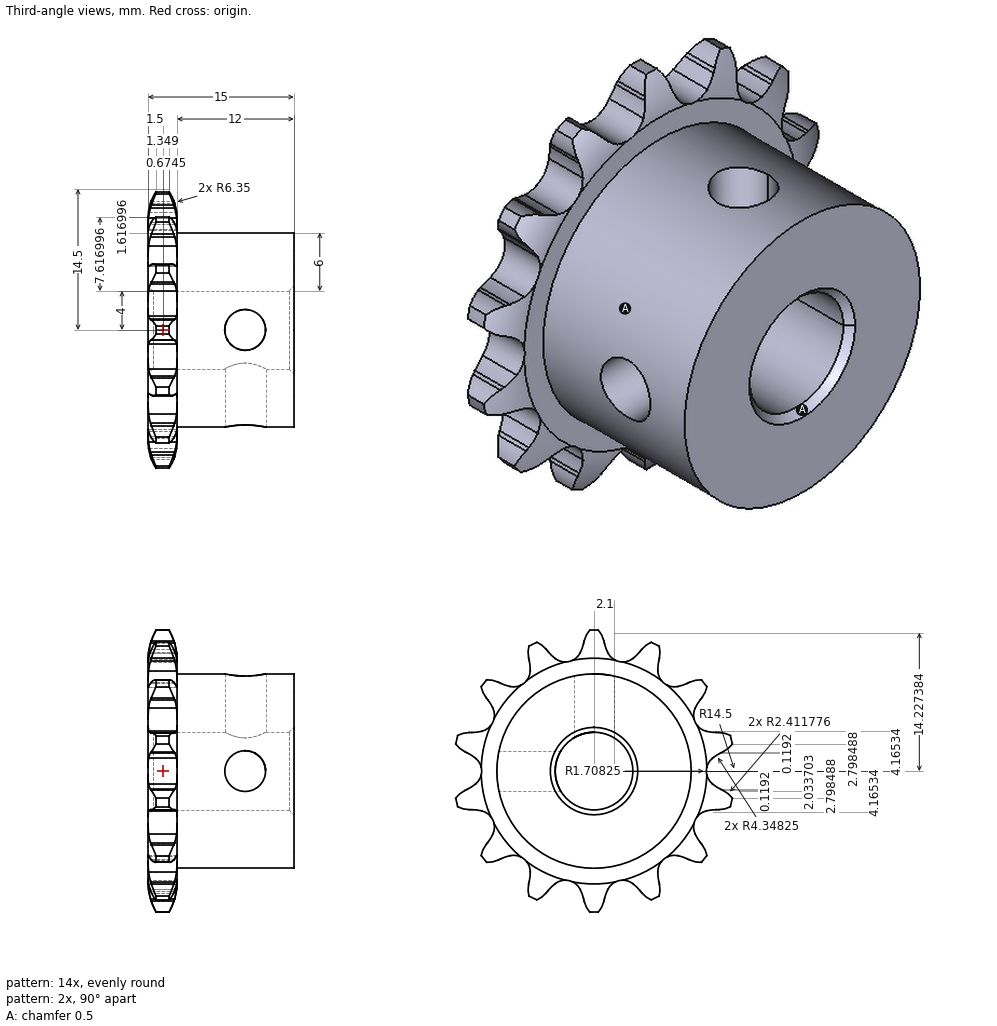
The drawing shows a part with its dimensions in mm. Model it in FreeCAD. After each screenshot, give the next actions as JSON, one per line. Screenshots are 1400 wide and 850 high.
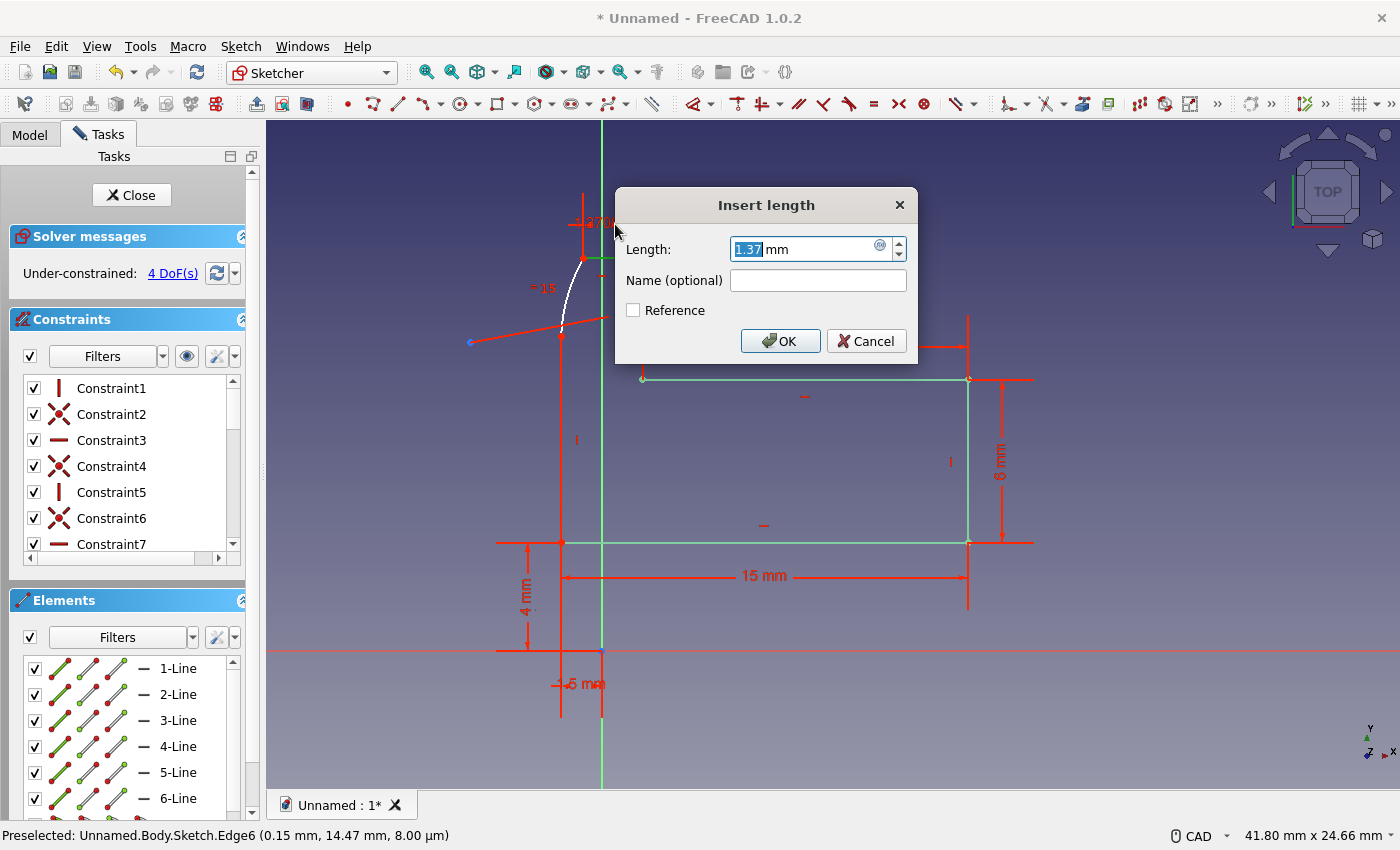
{"action": "type", "text": "1.349"}
{"action": "key", "text": "Return"}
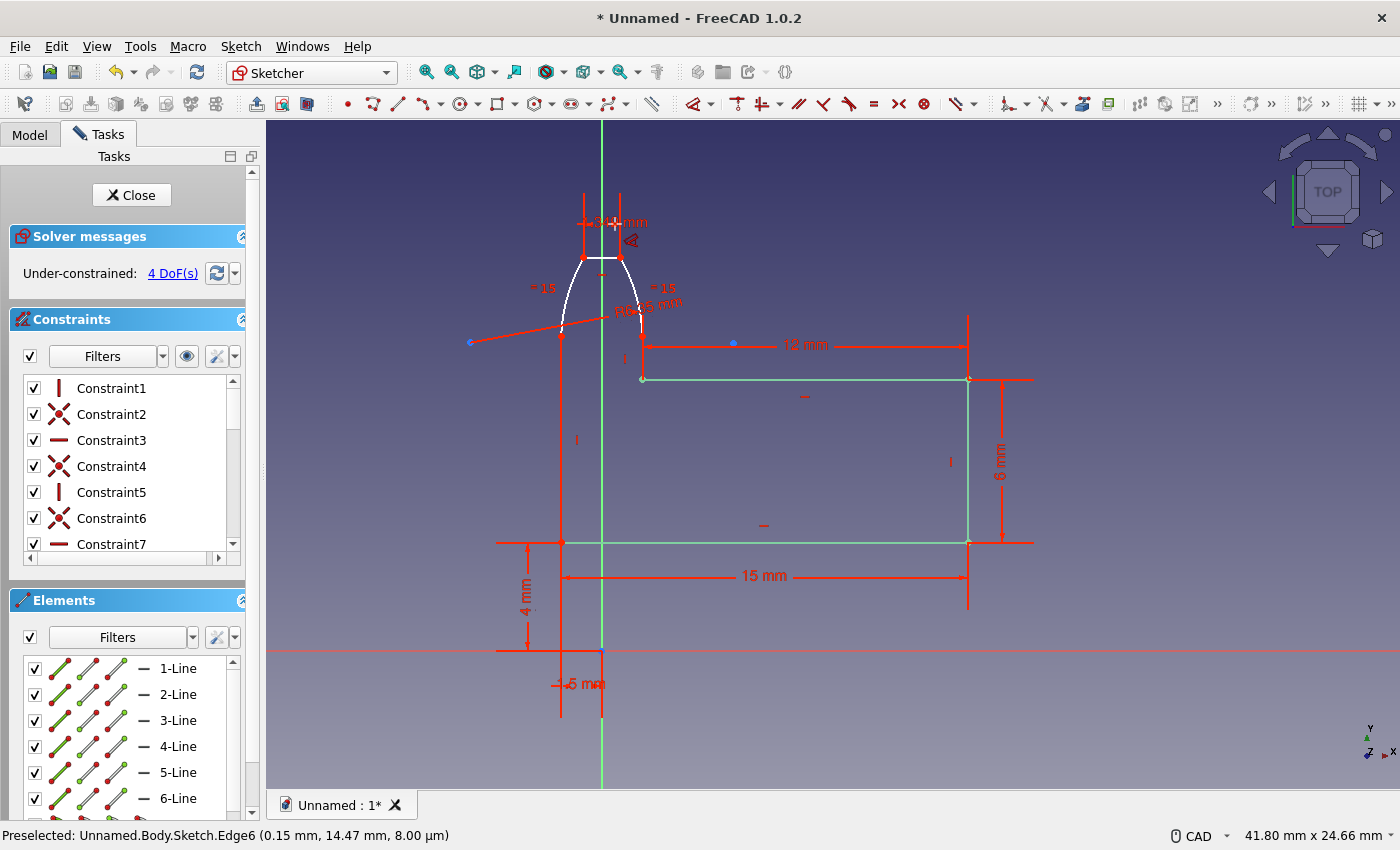
{"action": "left_click", "coordinate": [620, 258]}
{"action": "left_click", "coordinate": [654, 454]}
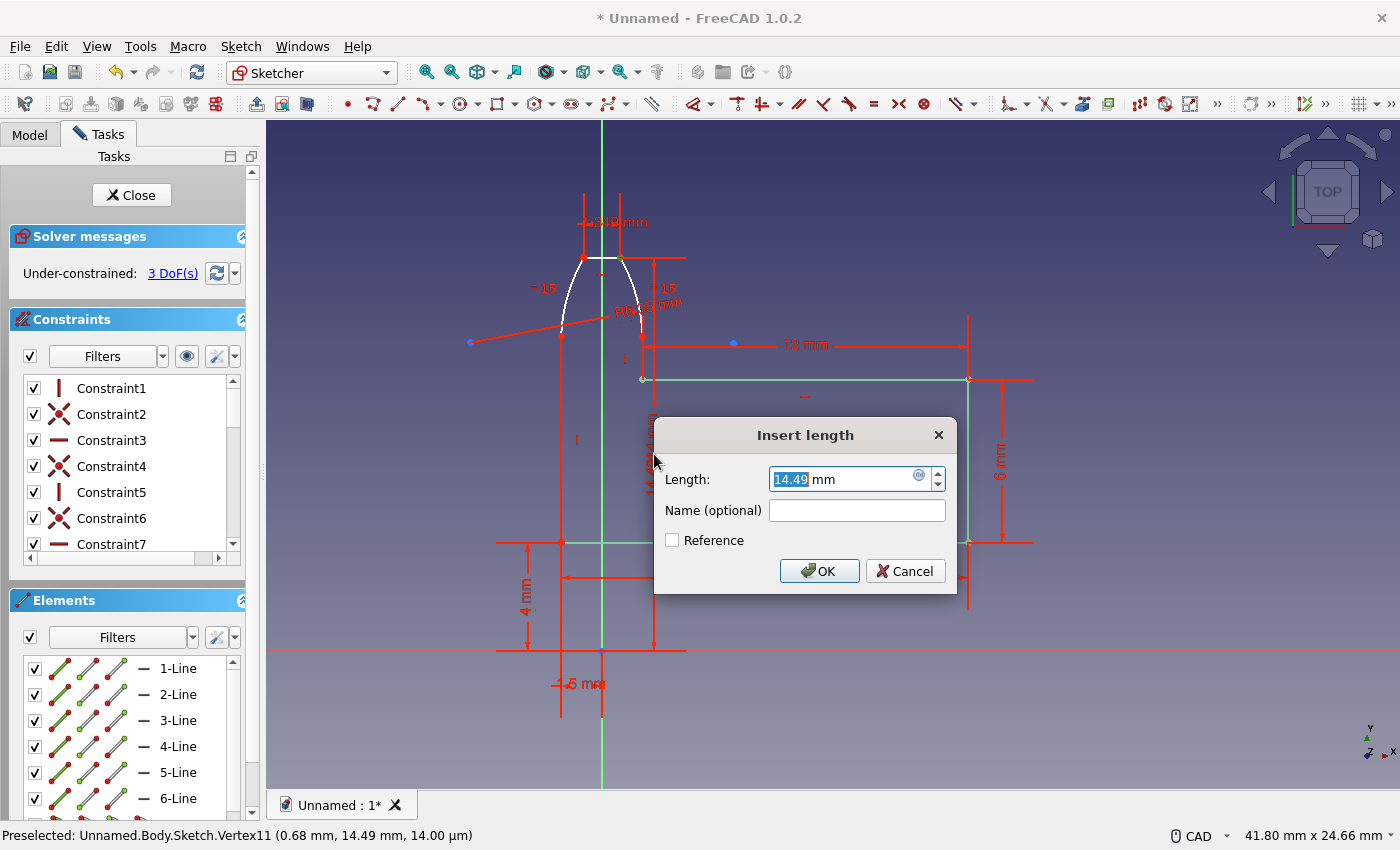
{"action": "type", "text": "14.5"}
{"action": "key", "text": "Return"}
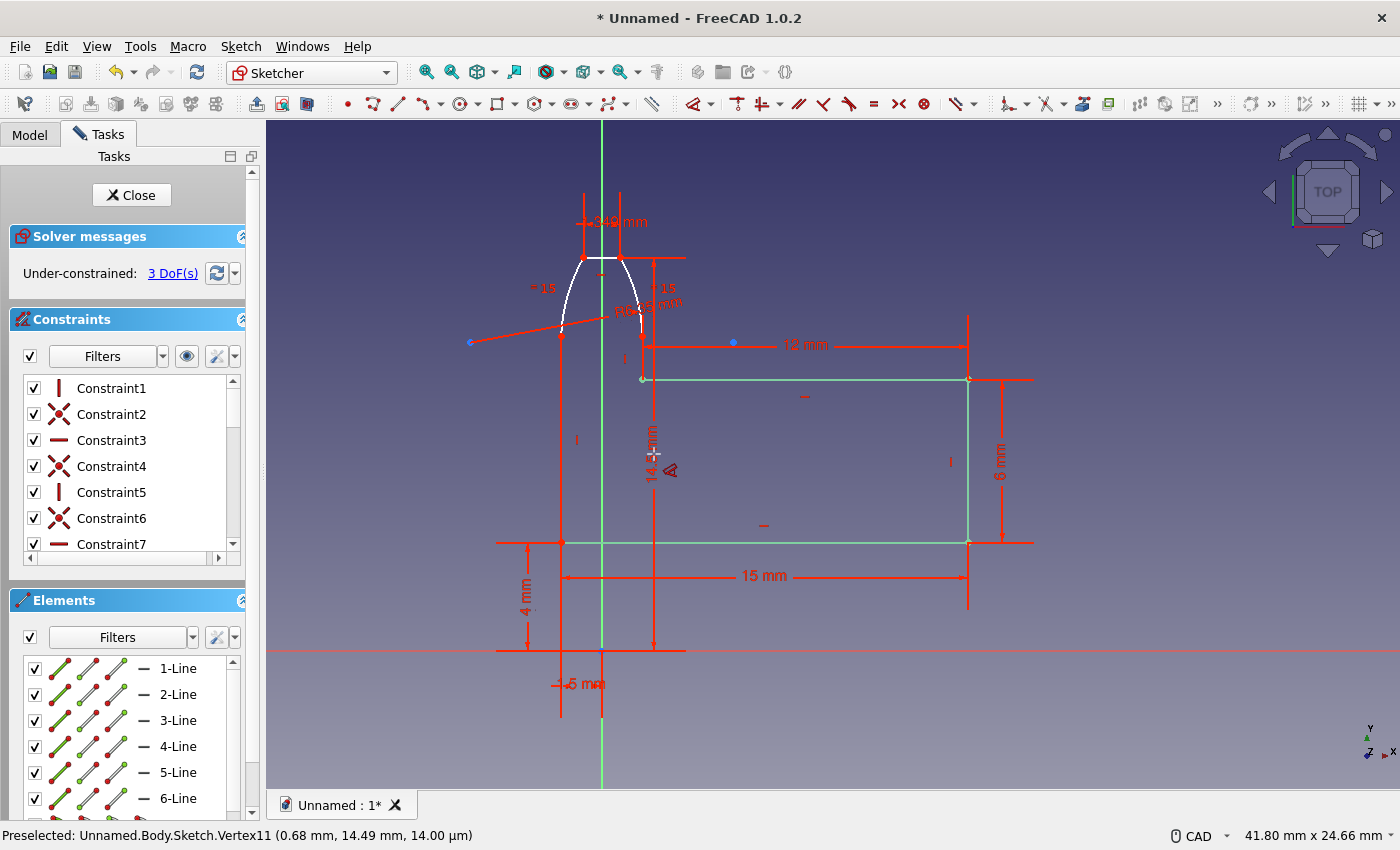
{"action": "scroll", "coordinate": [620, 258], "scroll_direction": "up", "scroll_amount": 4}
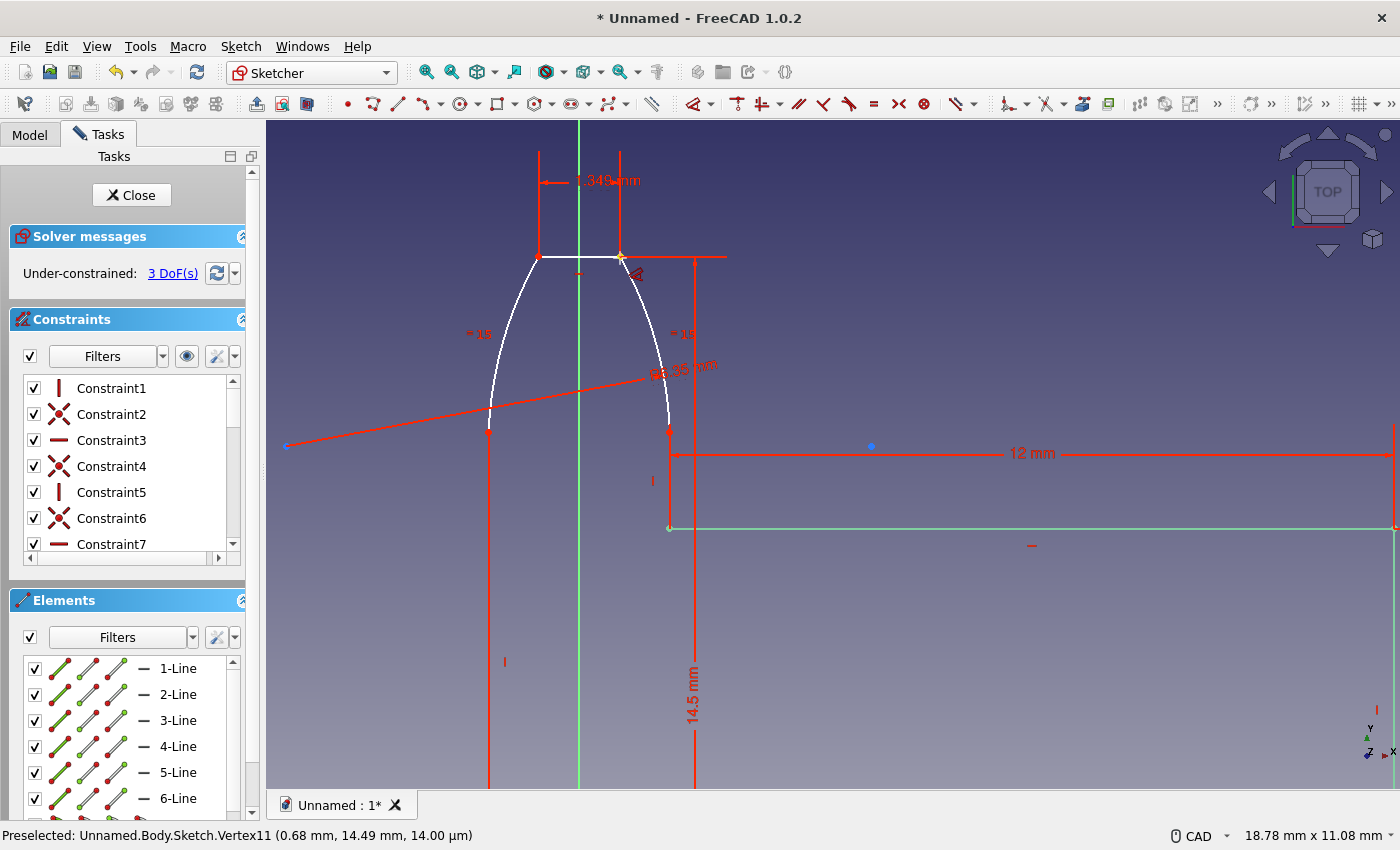
{"action": "left_click", "coordinate": [620, 257]}
{"action": "left_click", "coordinate": [600, 223]}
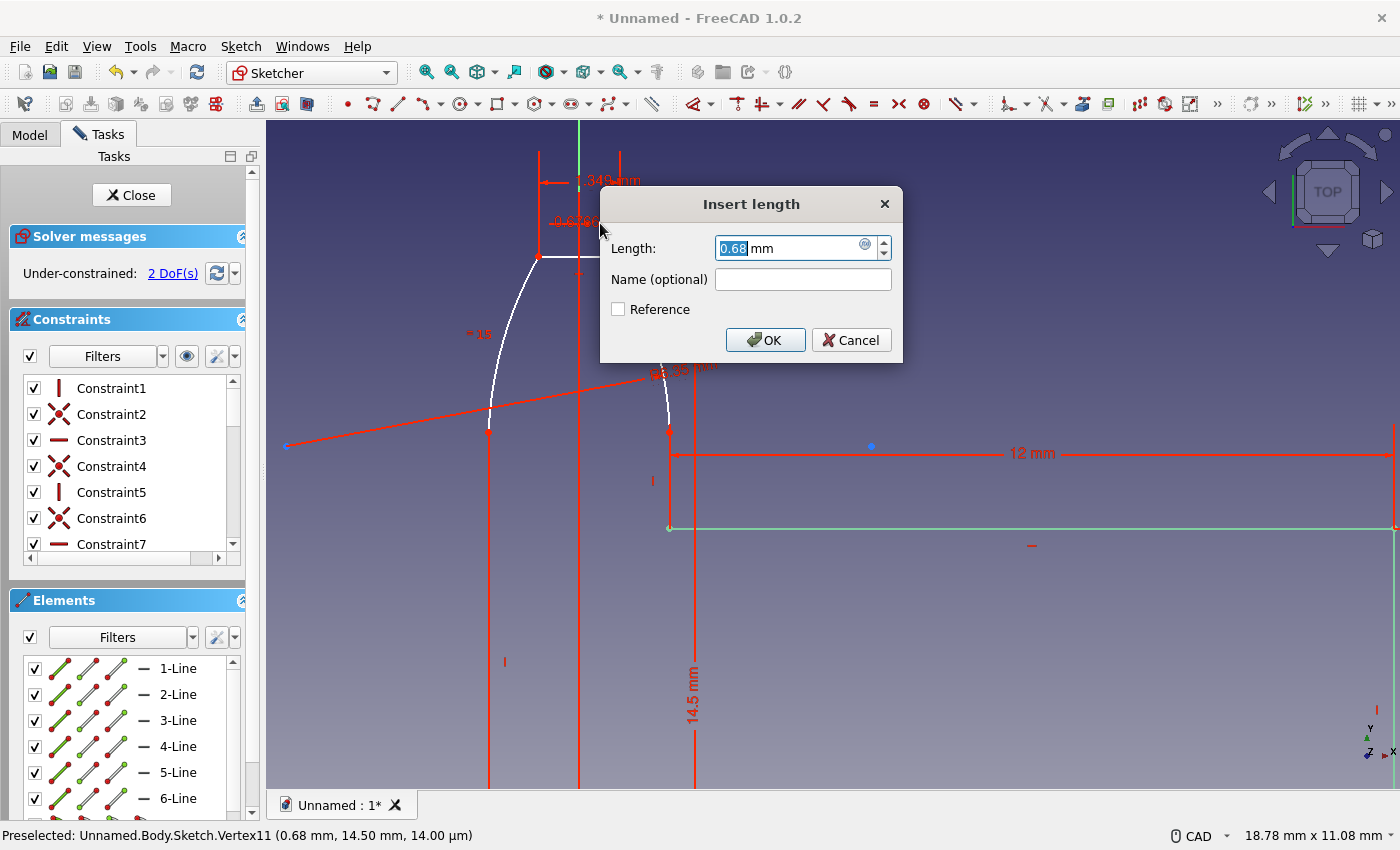
{"action": "type", "text": "0.6745"}
{"action": "key", "text": "Return"}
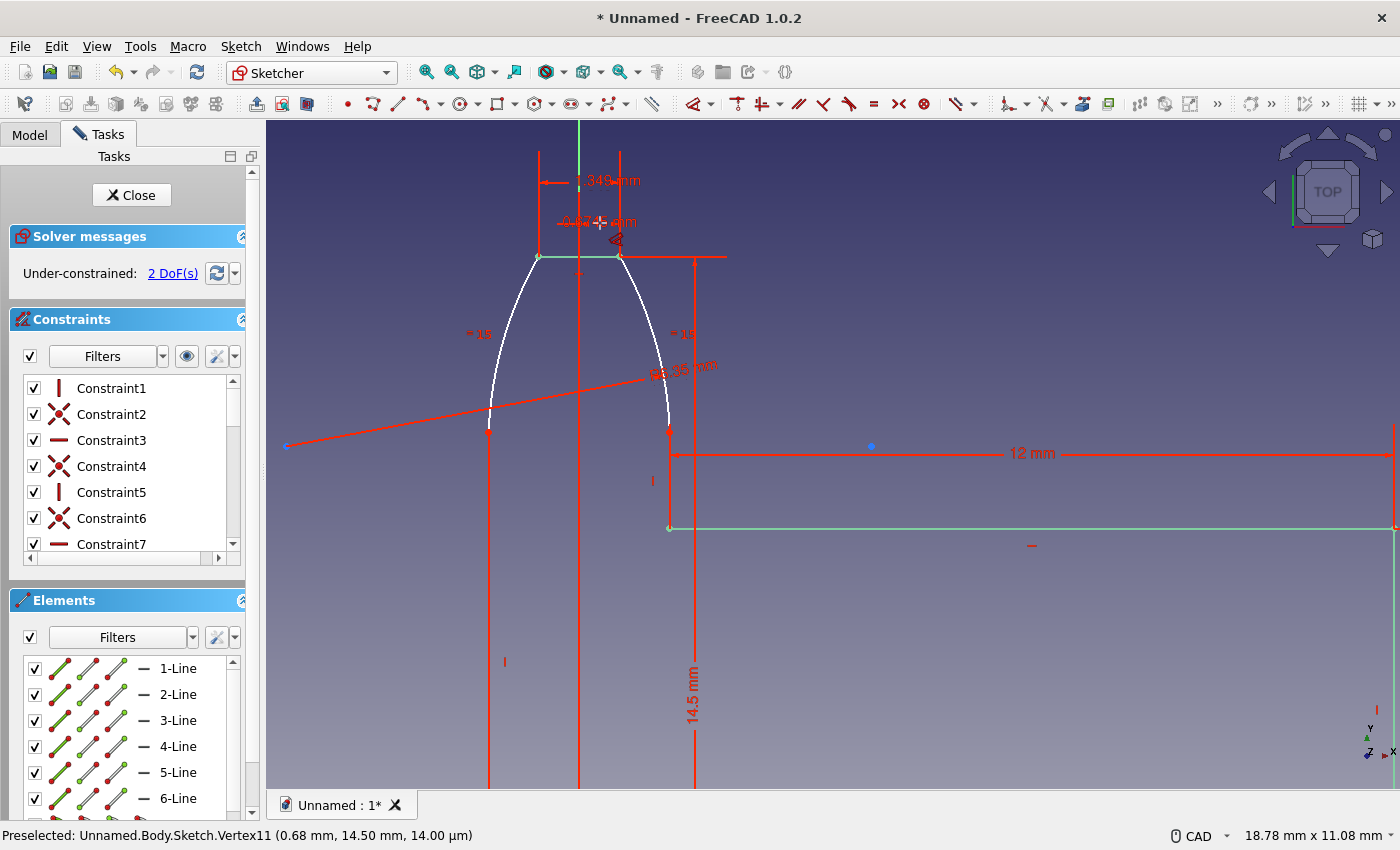
{"action": "left_click", "coordinate": [489, 570]}
{"action": "left_click", "coordinate": [455, 597]}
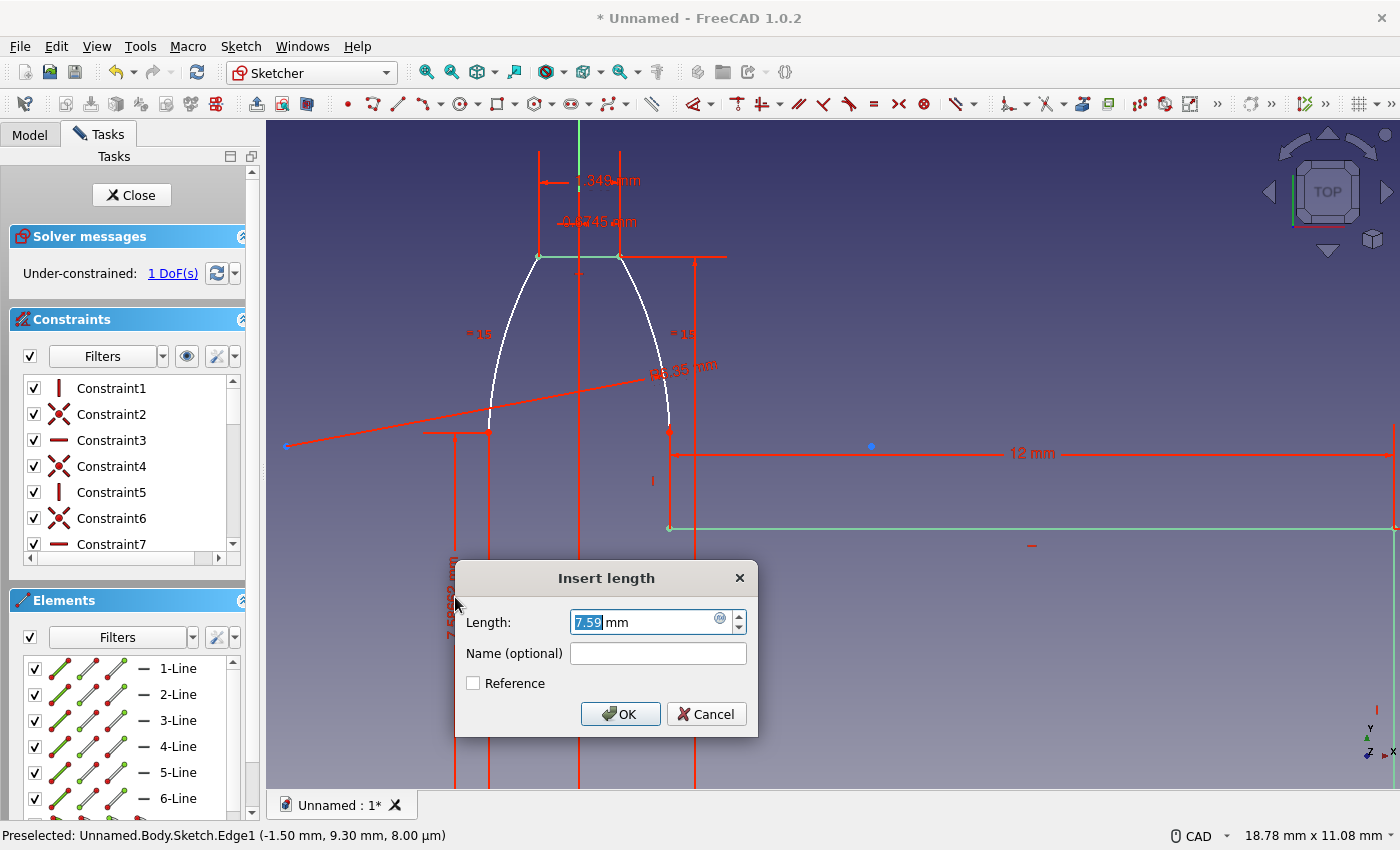
{"action": "type", "text": "7.616996"}
{"action": "key", "text": "Return"}